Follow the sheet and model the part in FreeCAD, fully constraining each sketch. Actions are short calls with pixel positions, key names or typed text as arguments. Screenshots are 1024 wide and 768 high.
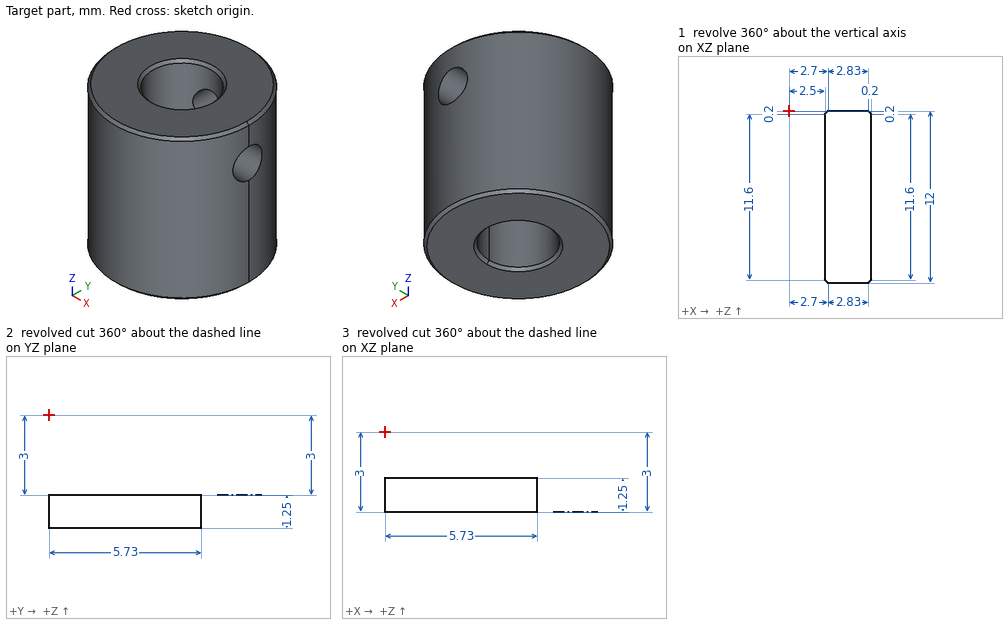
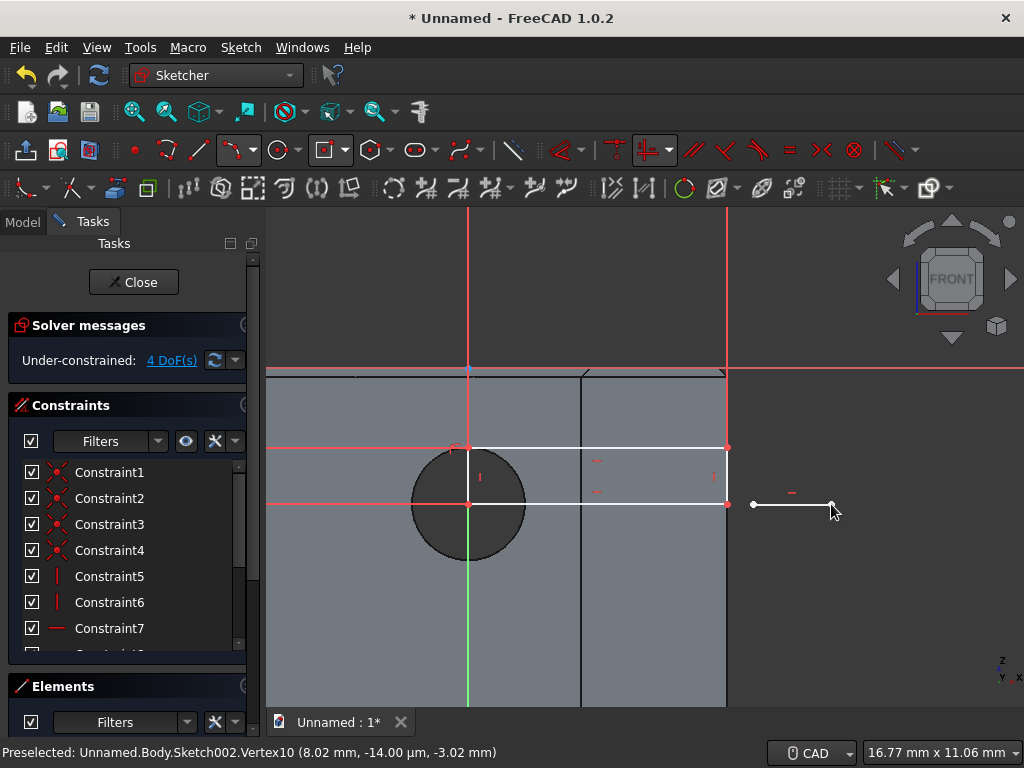
click(776, 505)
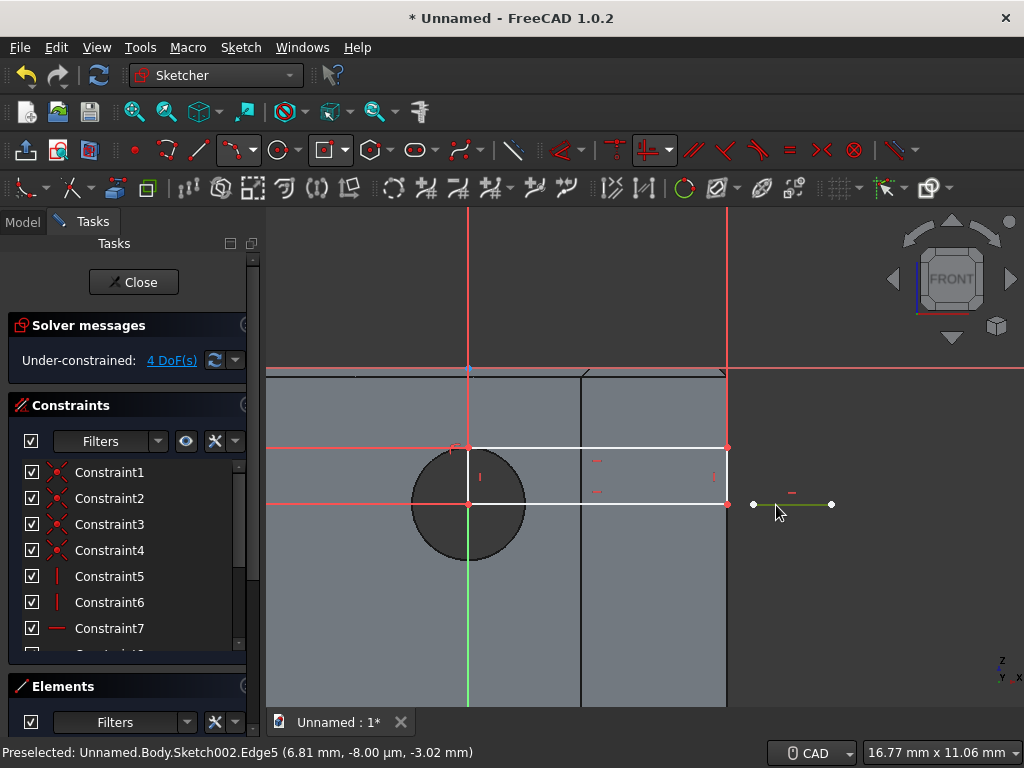
key(g)
key(n)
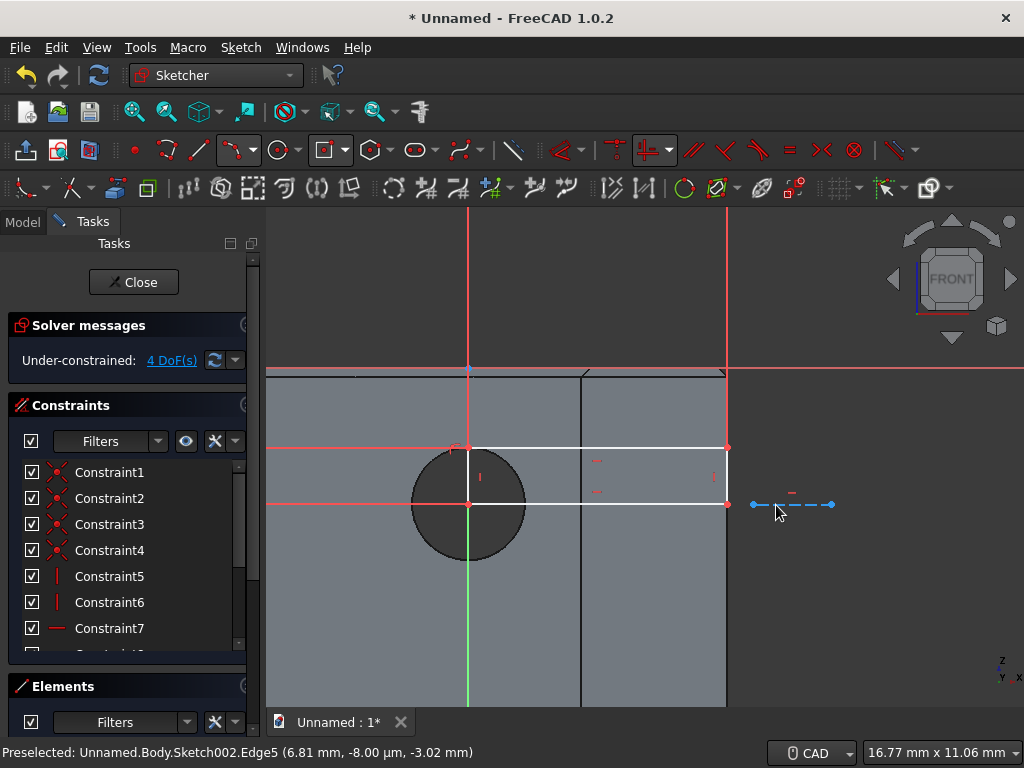
click(560, 150)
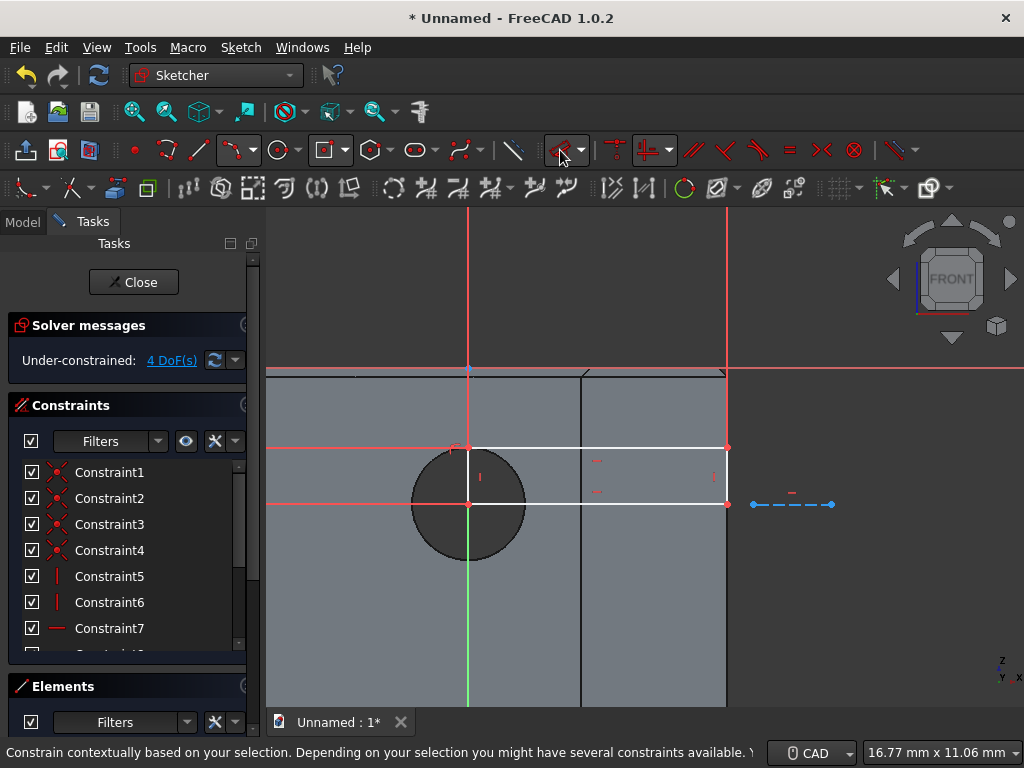
click(468, 504)
click(434, 436)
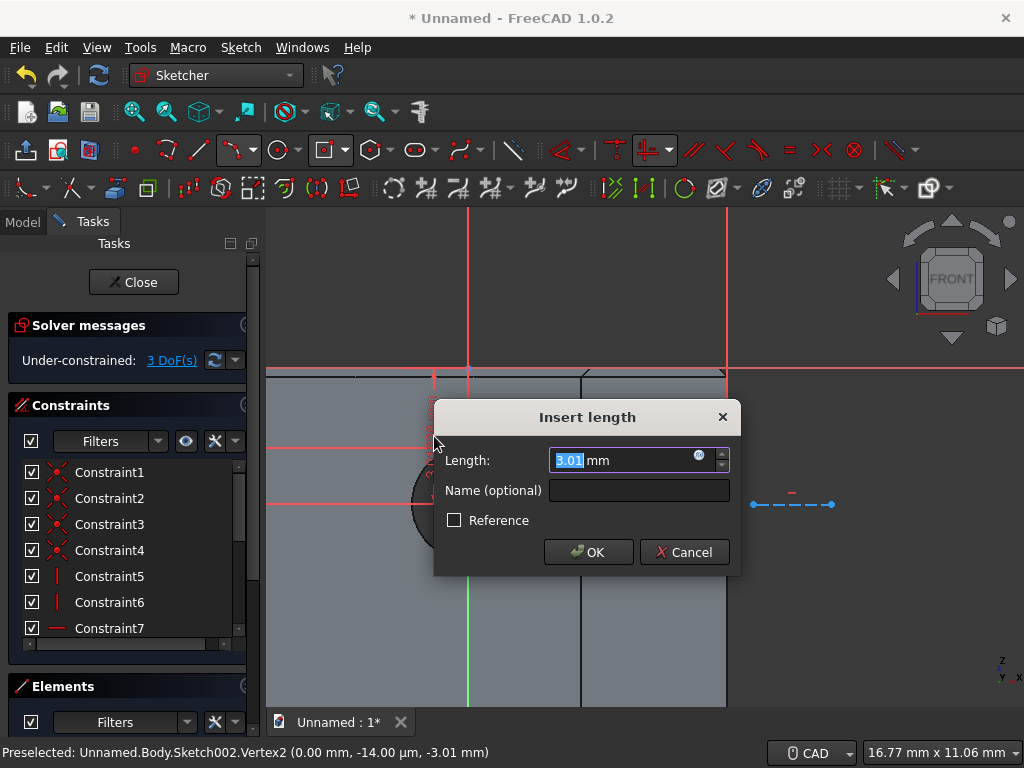
text(3)
key(Return)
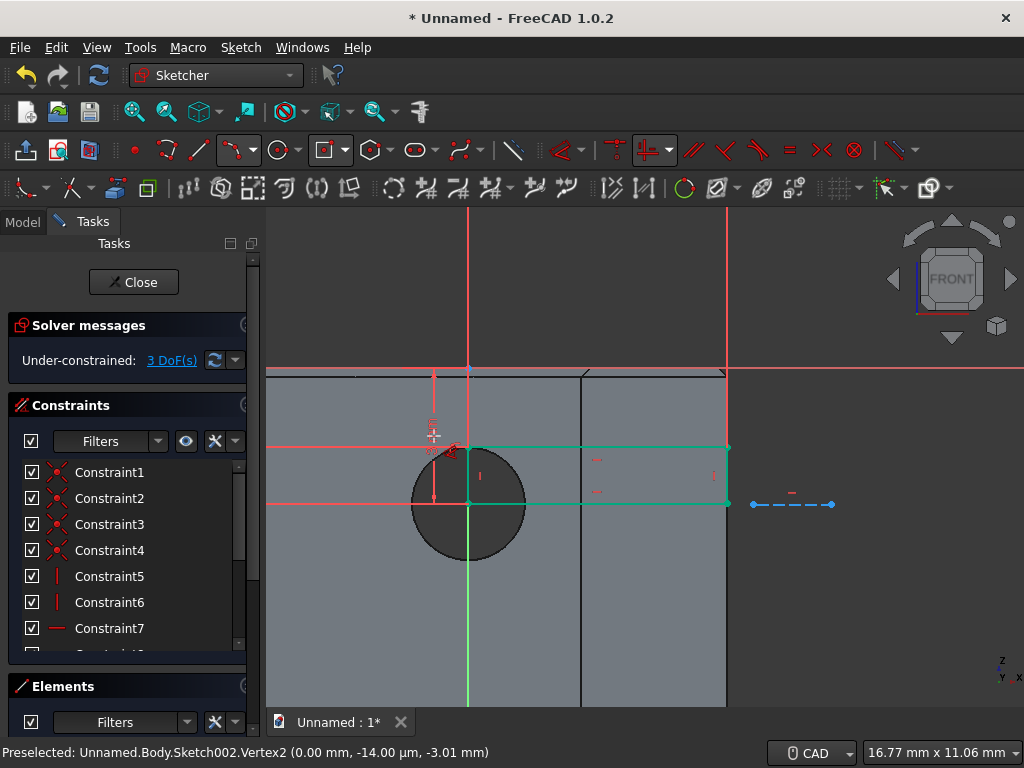
click(753, 505)
click(434, 405)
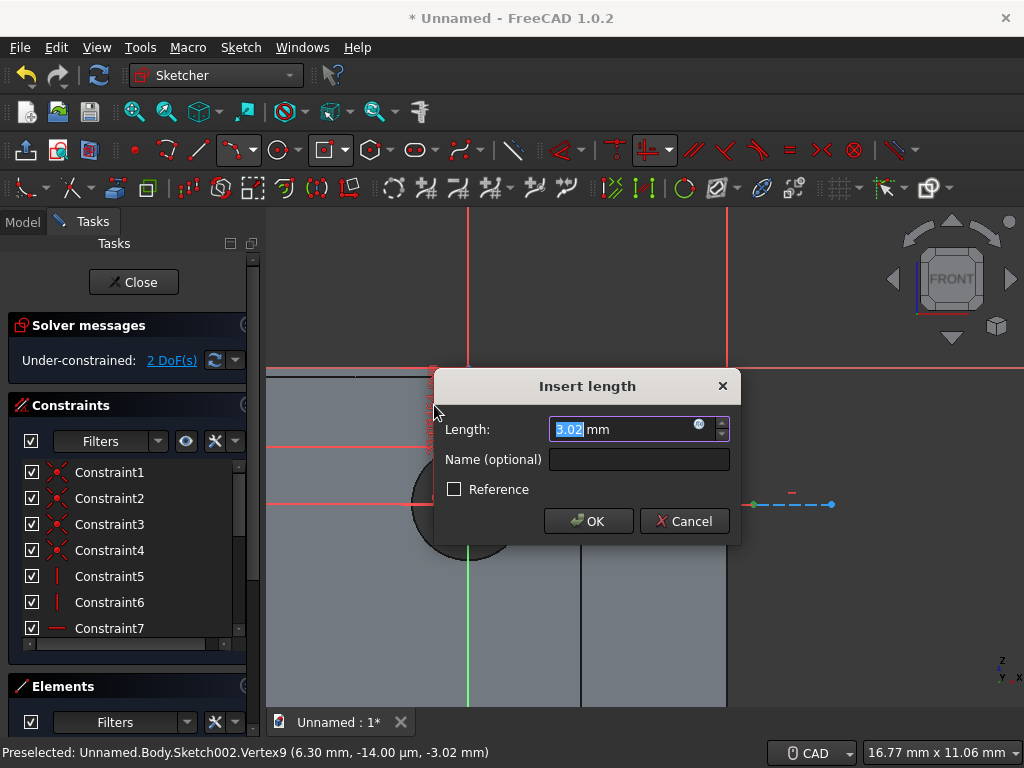
text(3)
key(Return)
key(Escape)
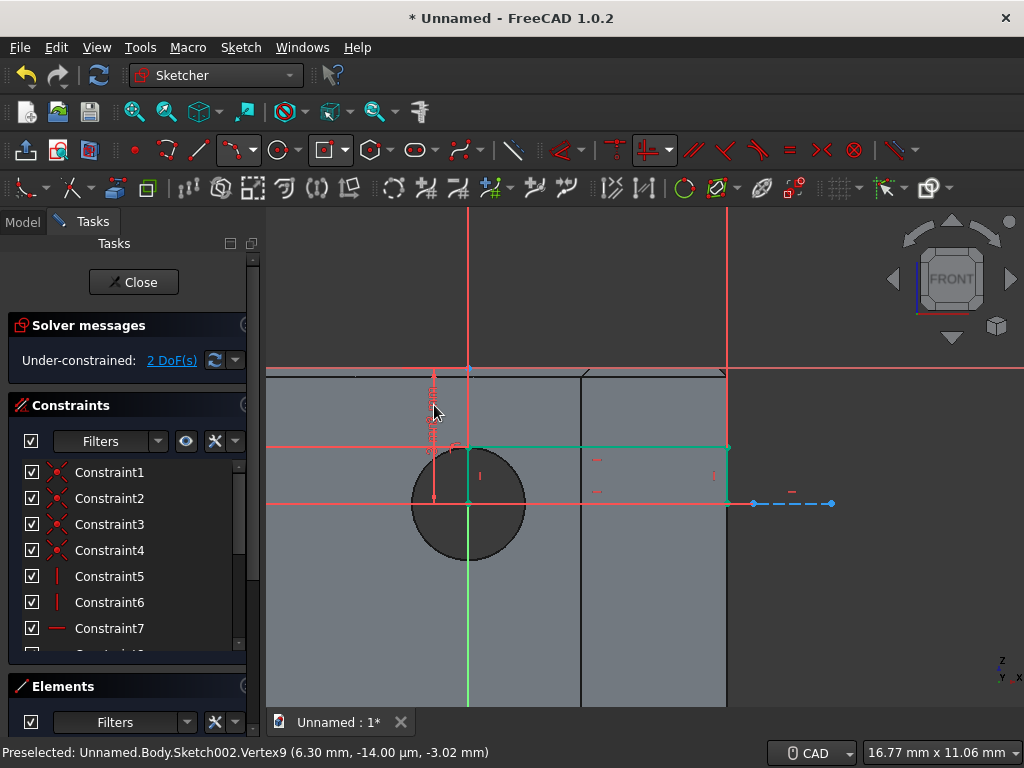
click(134, 282)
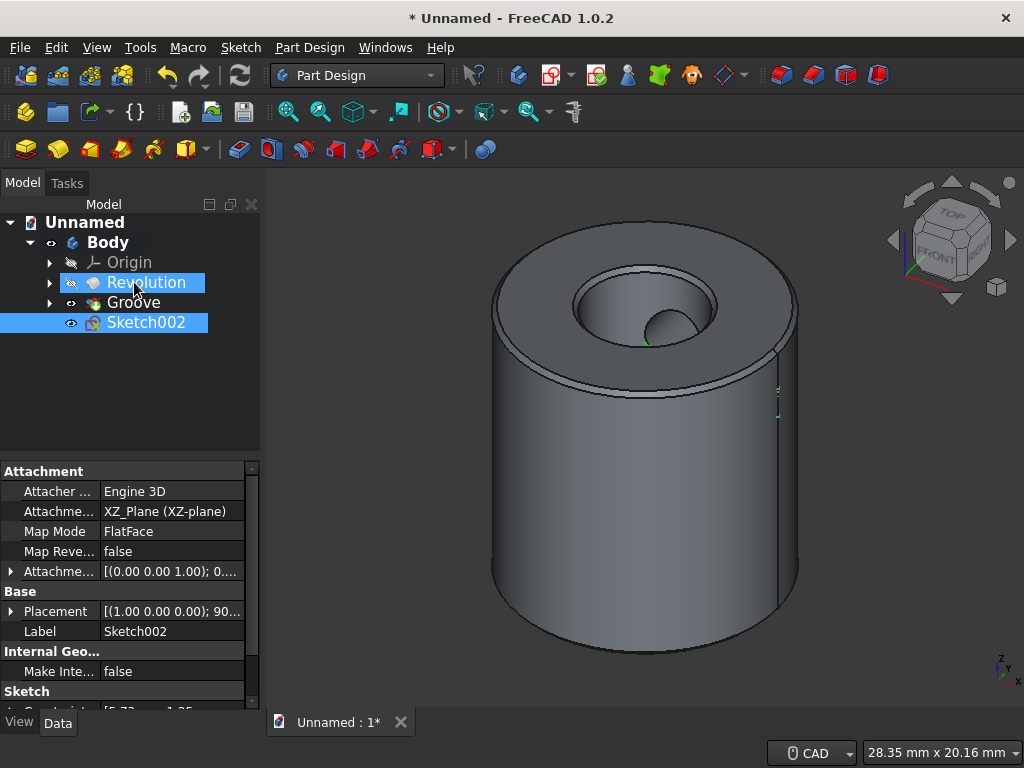
click(304, 150)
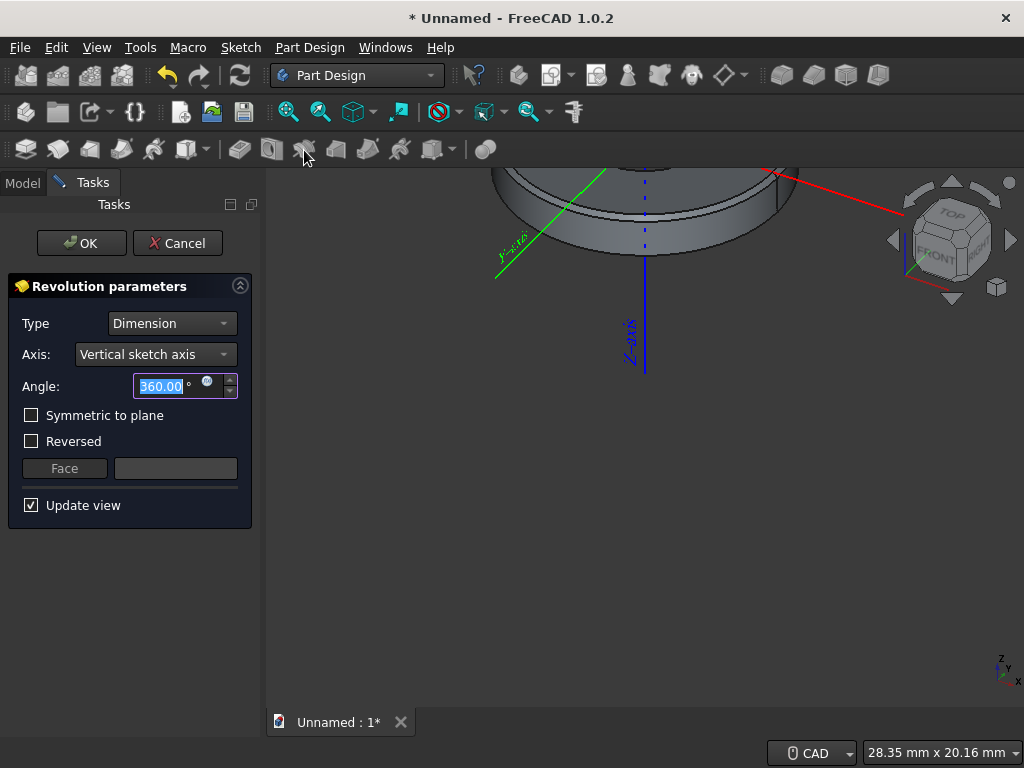
click(156, 354)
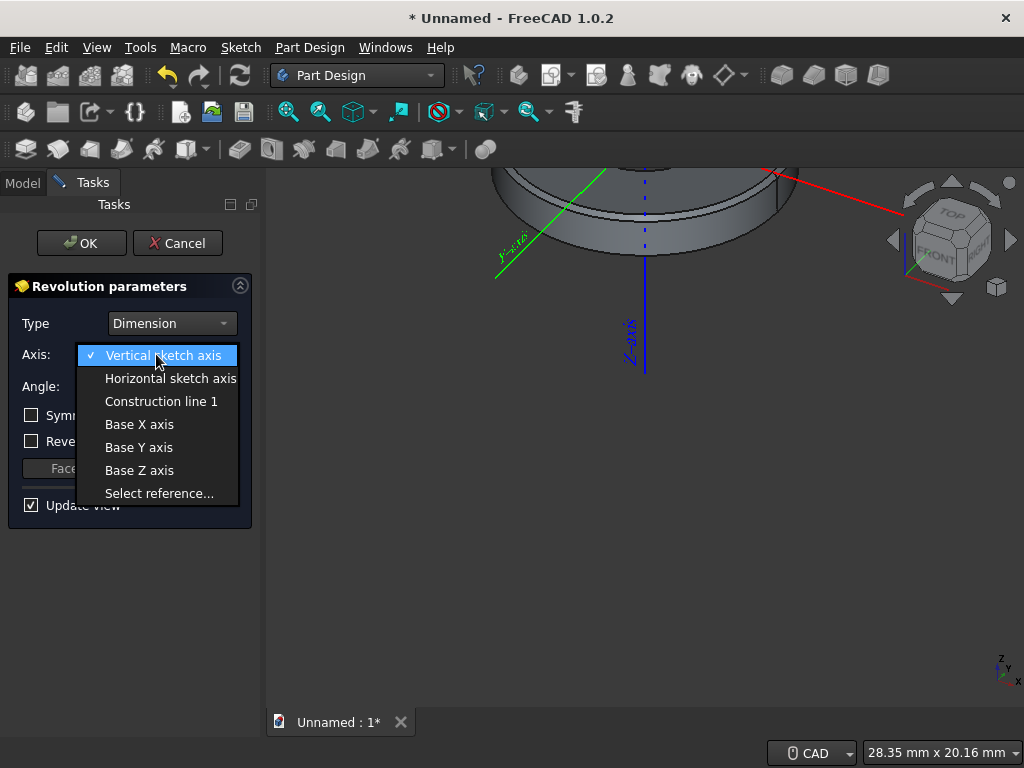
click(156, 402)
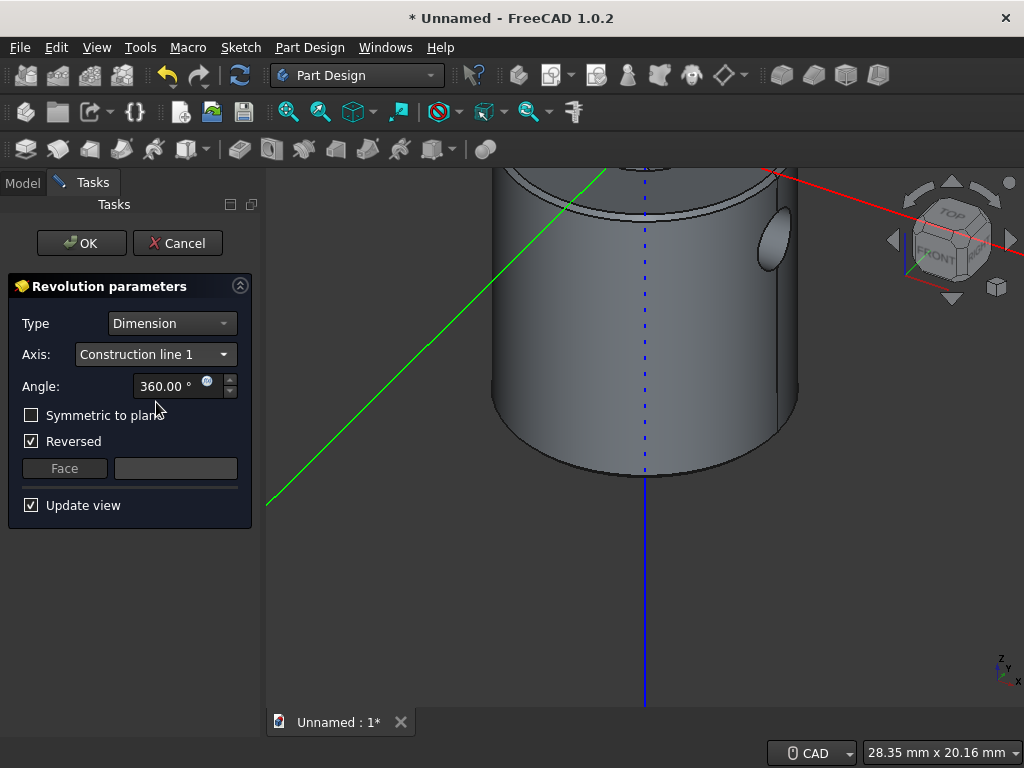
click(82, 243)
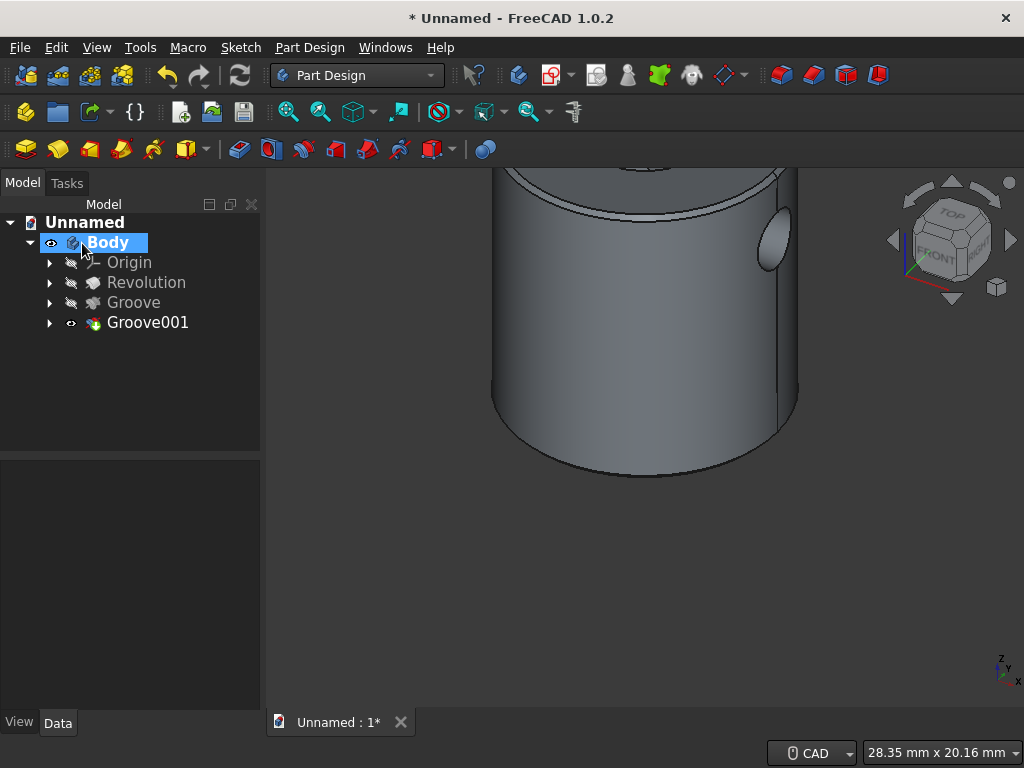
key(0)